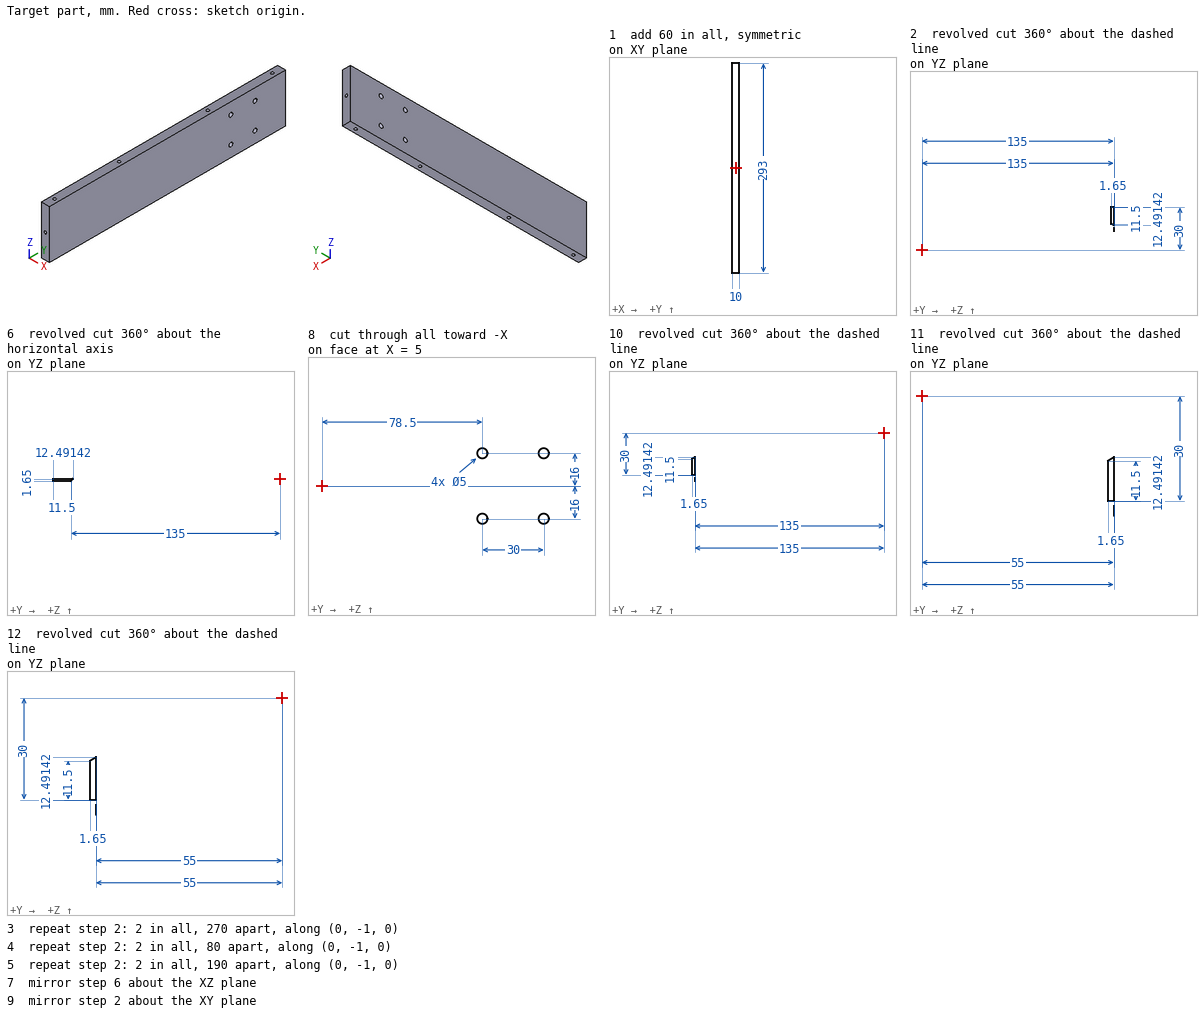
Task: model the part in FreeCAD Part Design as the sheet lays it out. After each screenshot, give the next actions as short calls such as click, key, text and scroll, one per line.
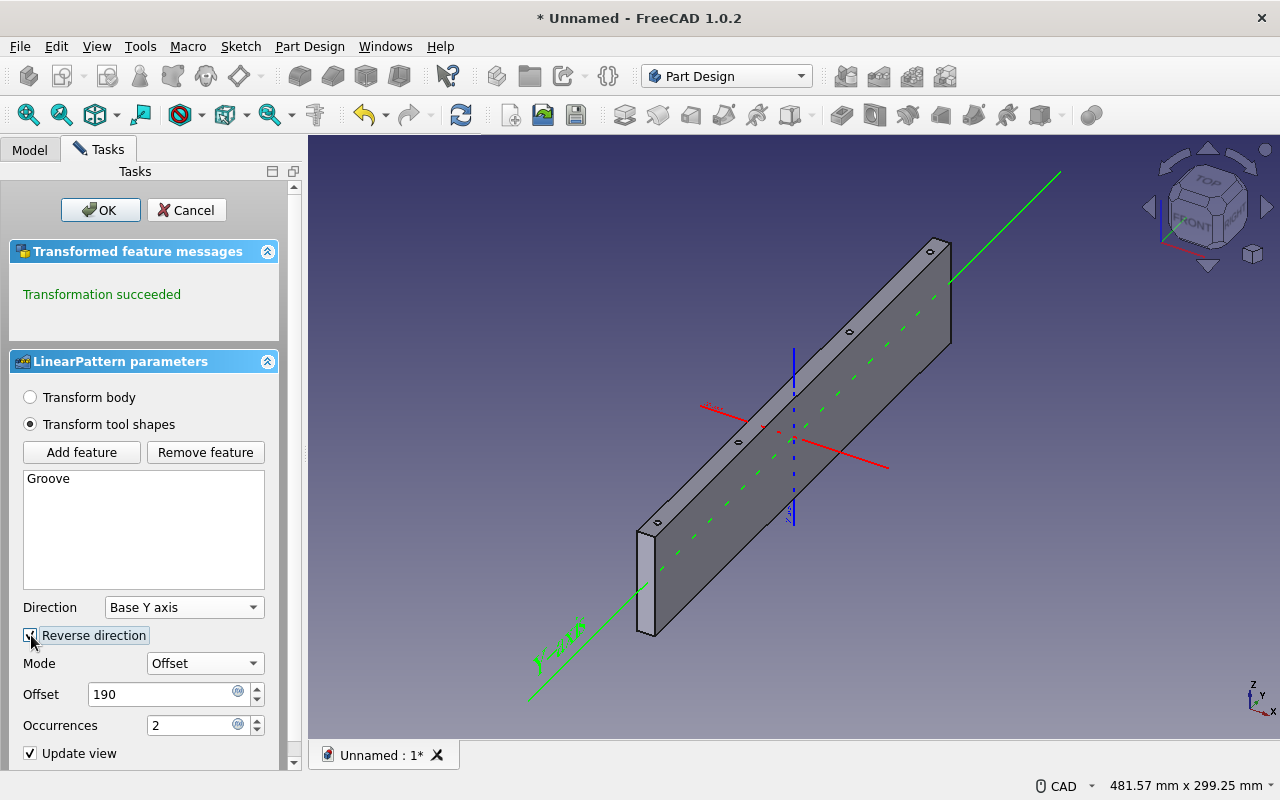
click(101, 210)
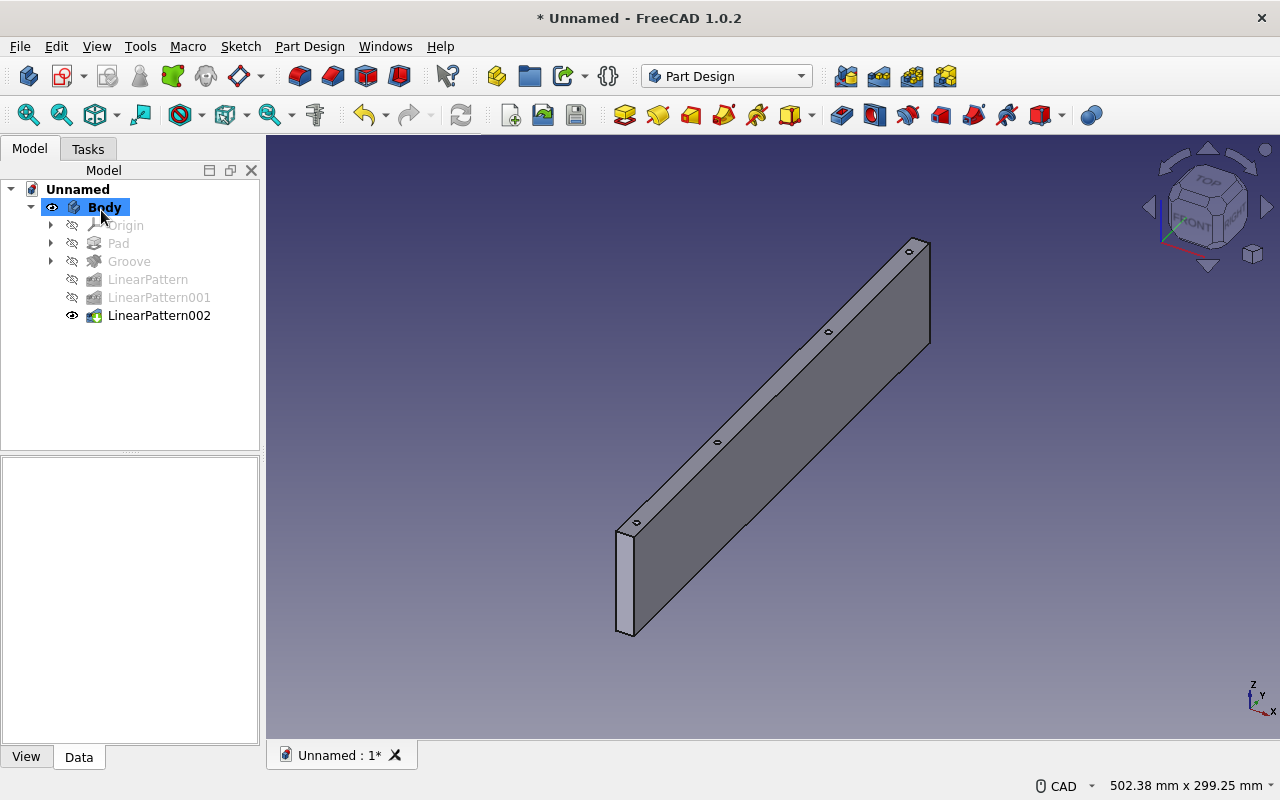
click(62, 76)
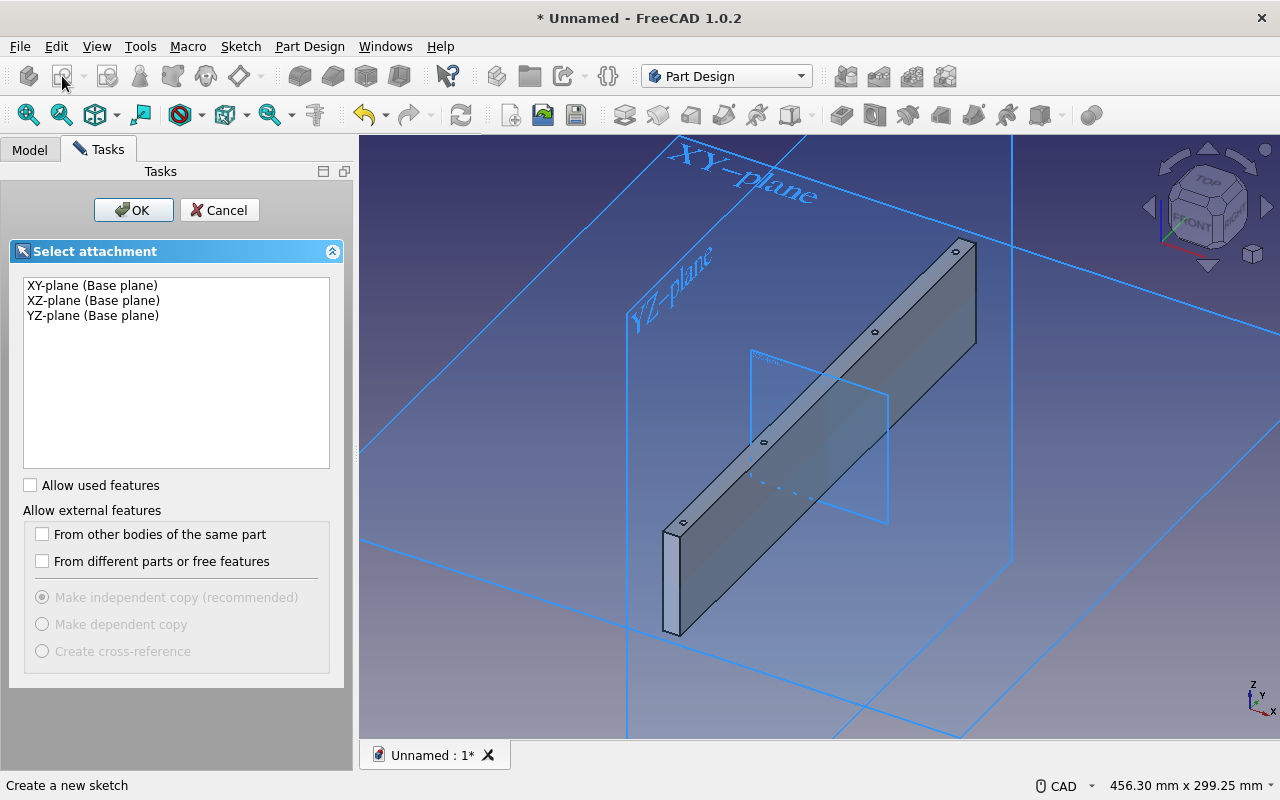
click(84, 316)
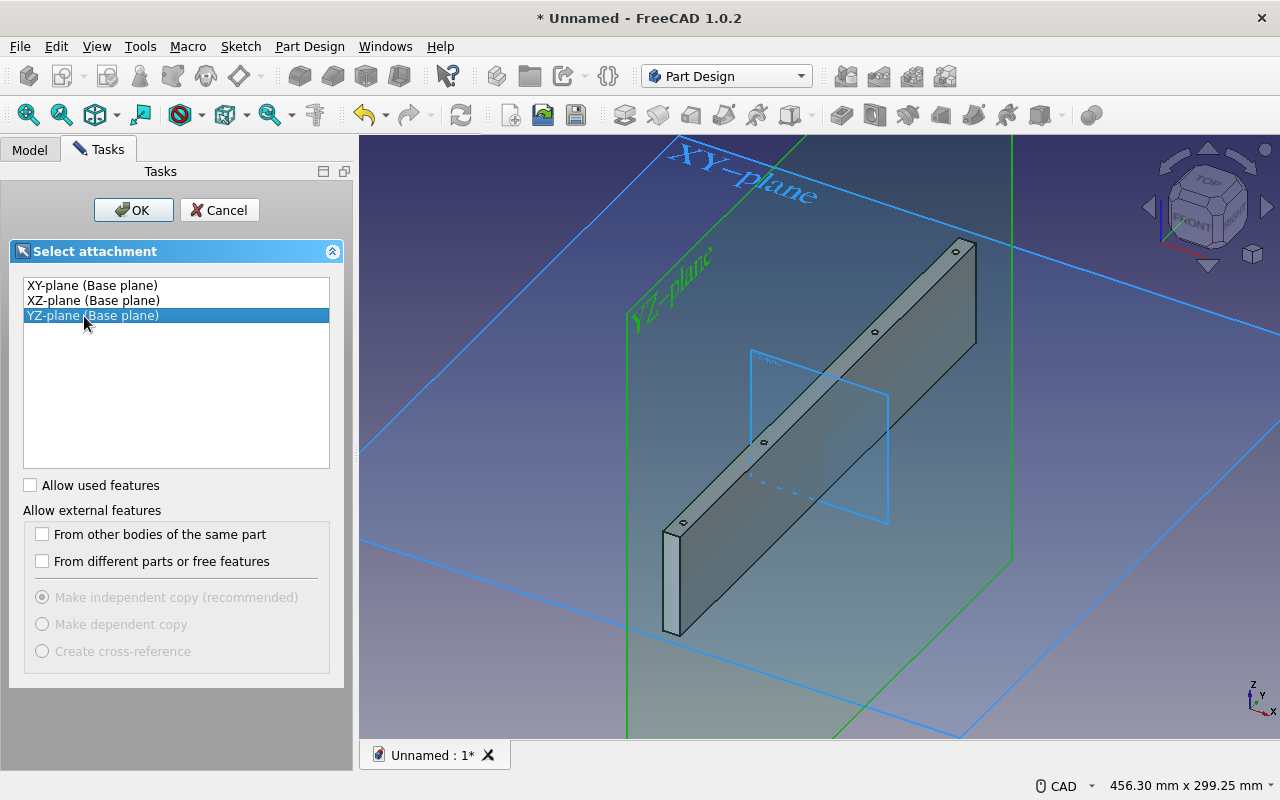
click(134, 210)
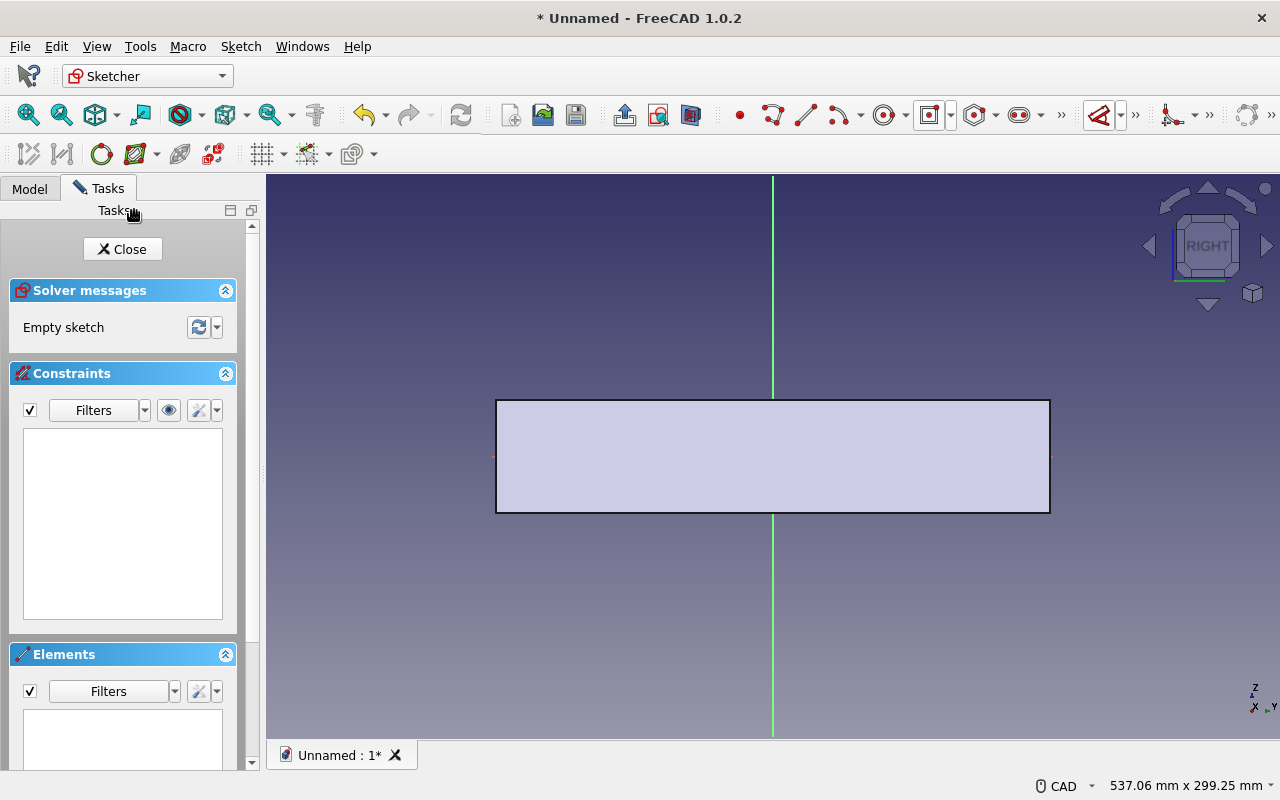
click(691, 116)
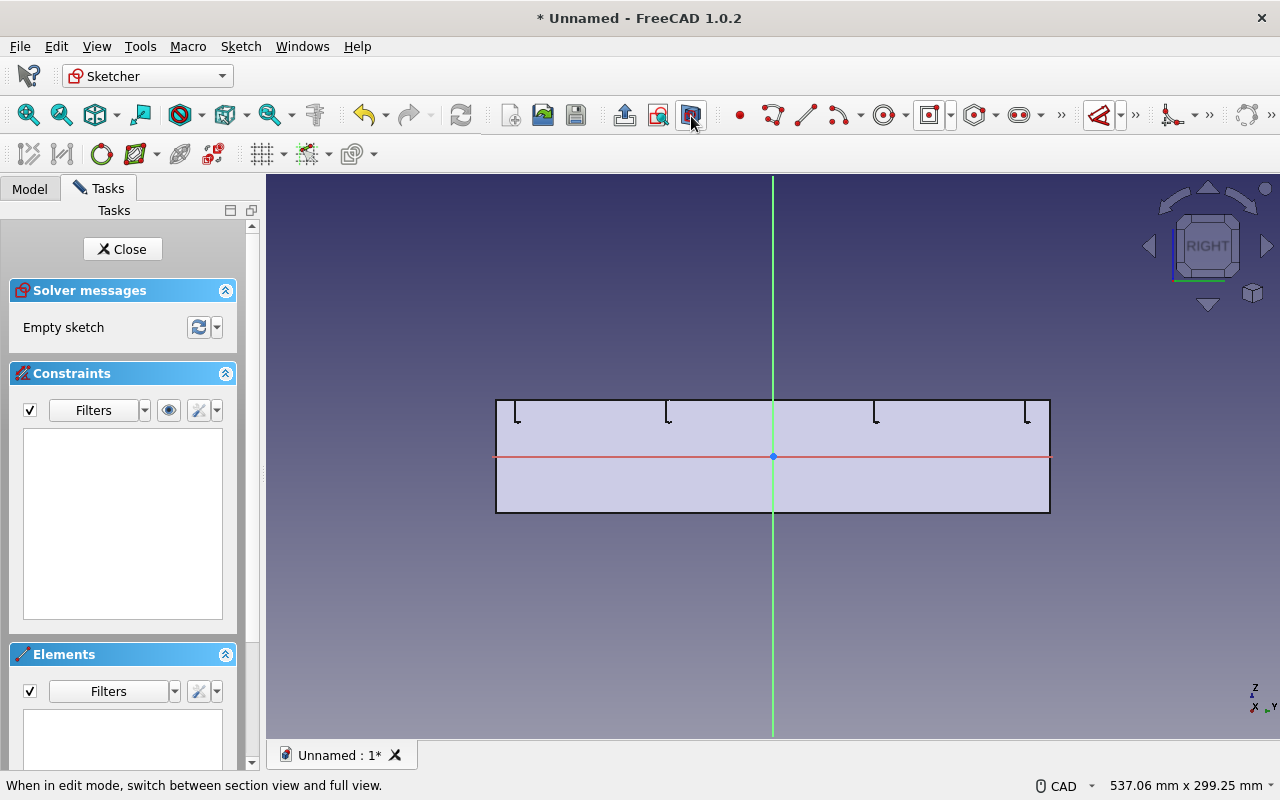
scroll(498, 458, up, 15)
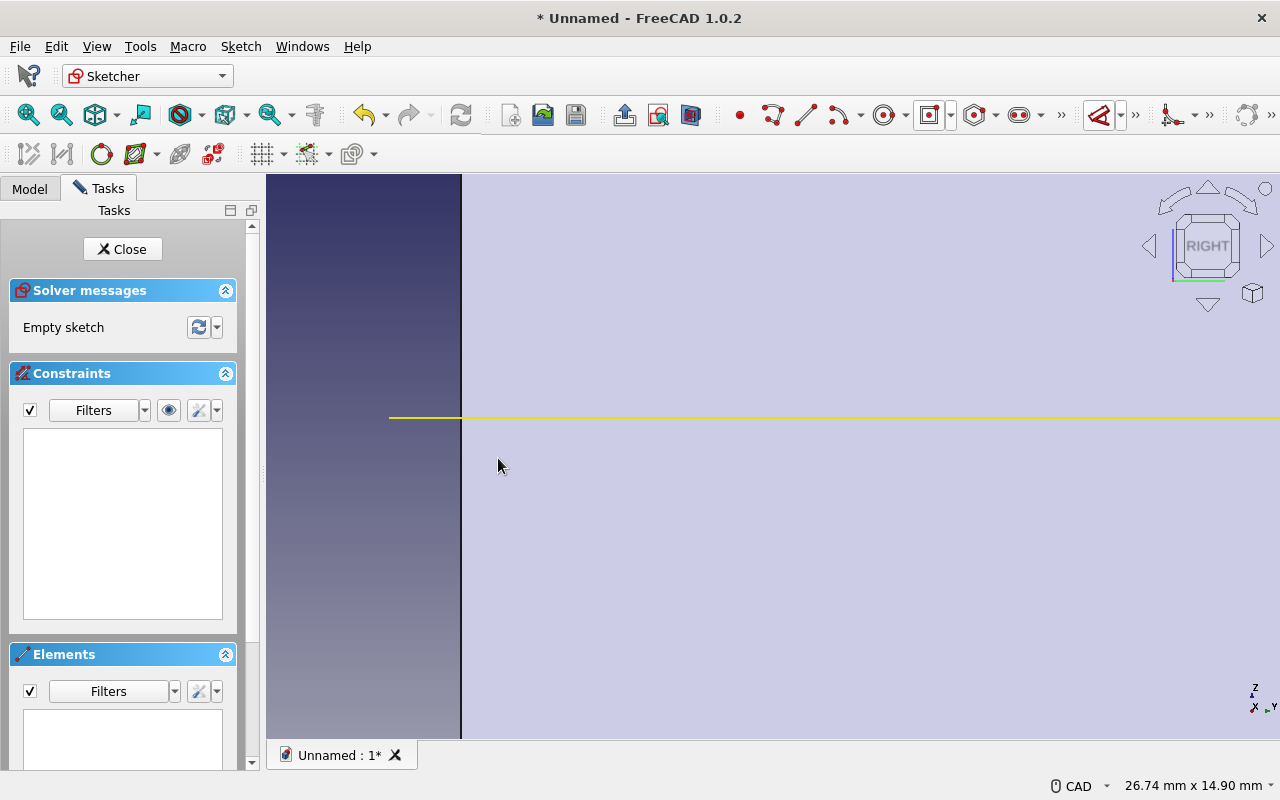
click(773, 116)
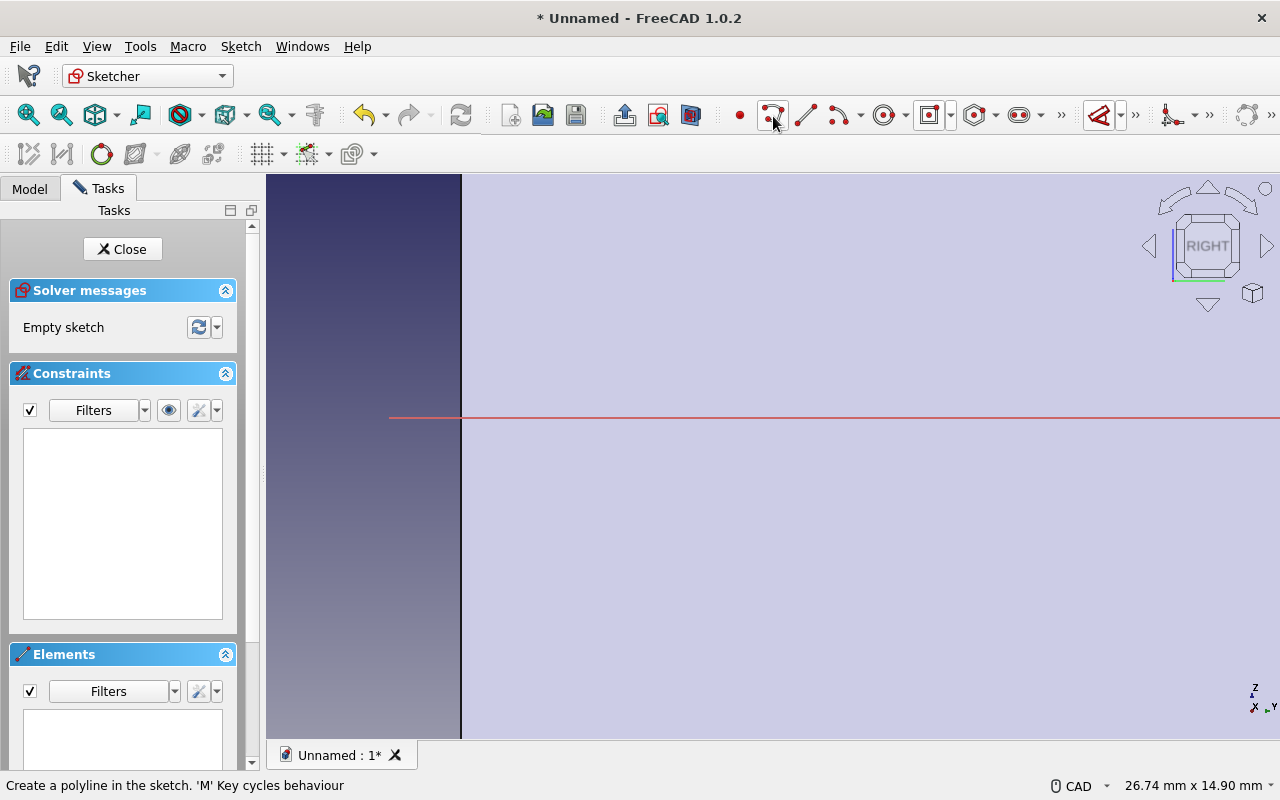
click(935, 418)
click(461, 427)
click(461, 481)
click(898, 481)
click(935, 418)
key(Escape)
key(Escape)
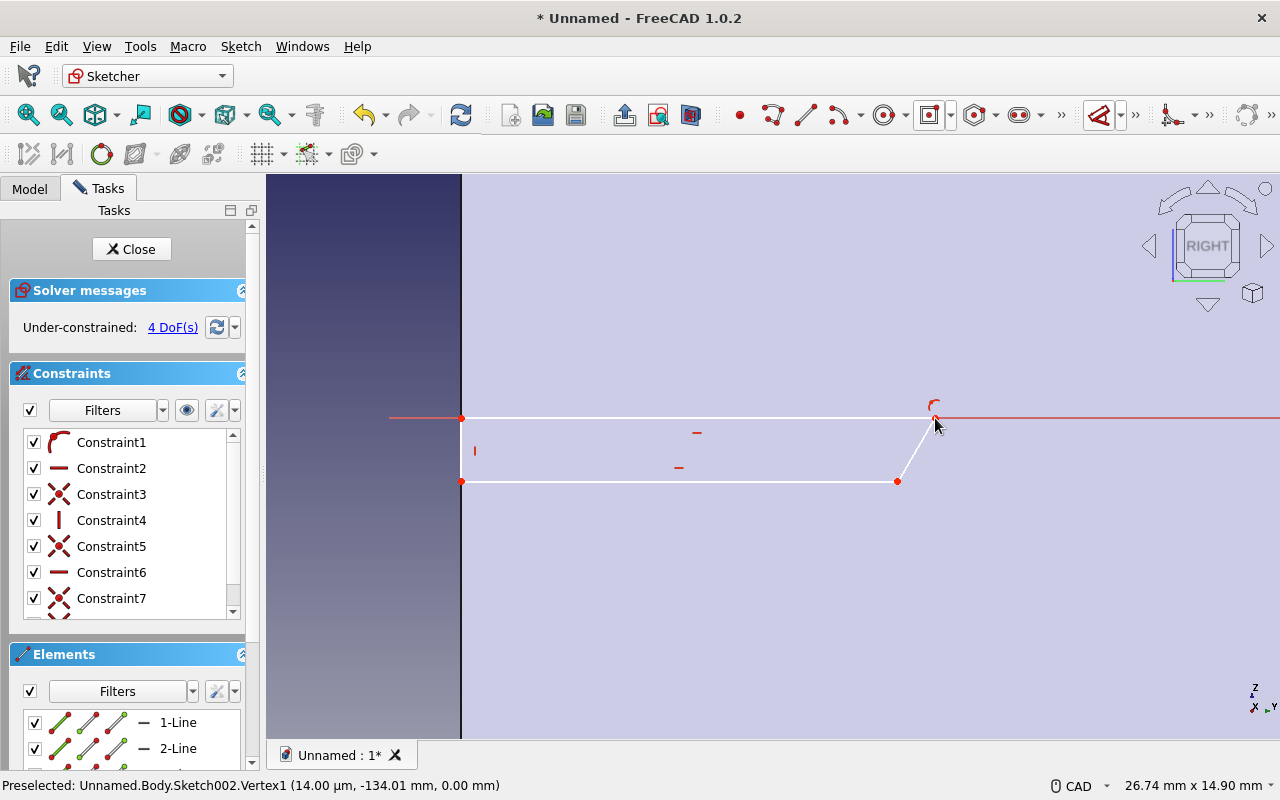
click(461, 437)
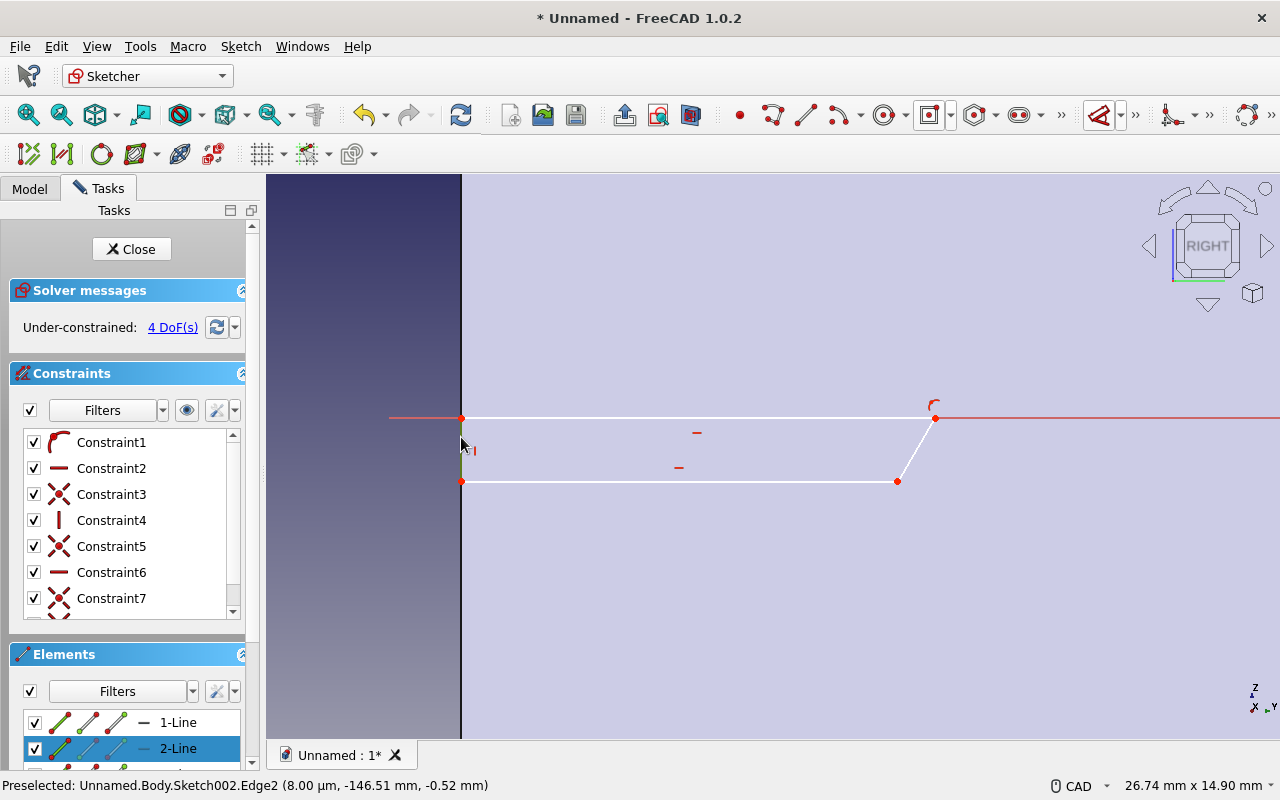
key(i)